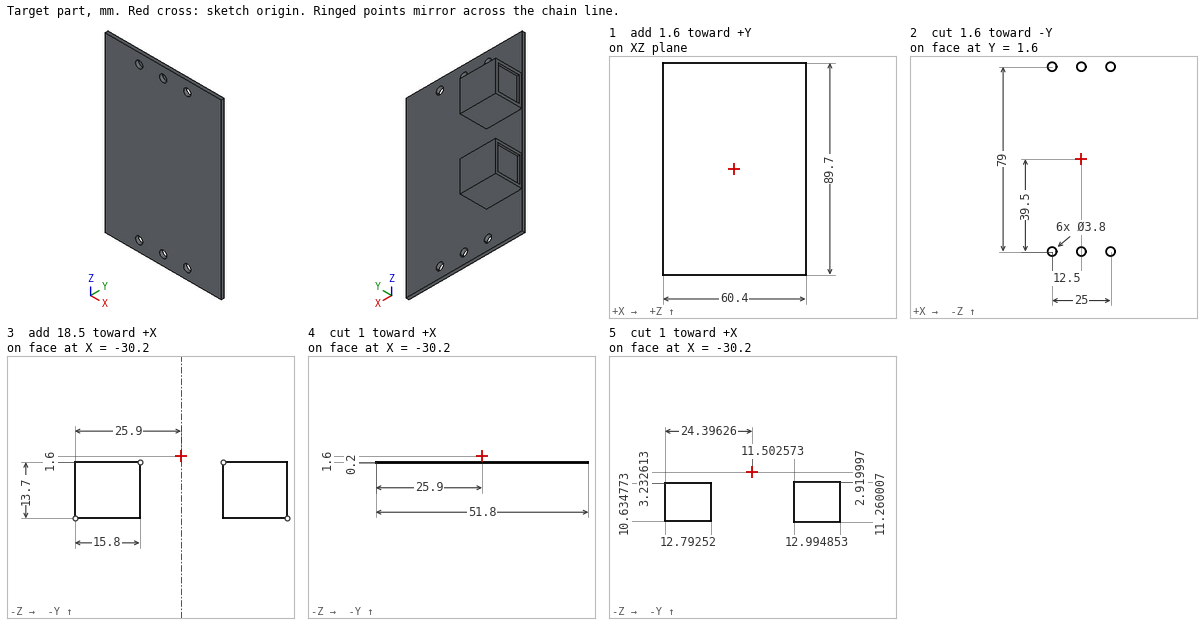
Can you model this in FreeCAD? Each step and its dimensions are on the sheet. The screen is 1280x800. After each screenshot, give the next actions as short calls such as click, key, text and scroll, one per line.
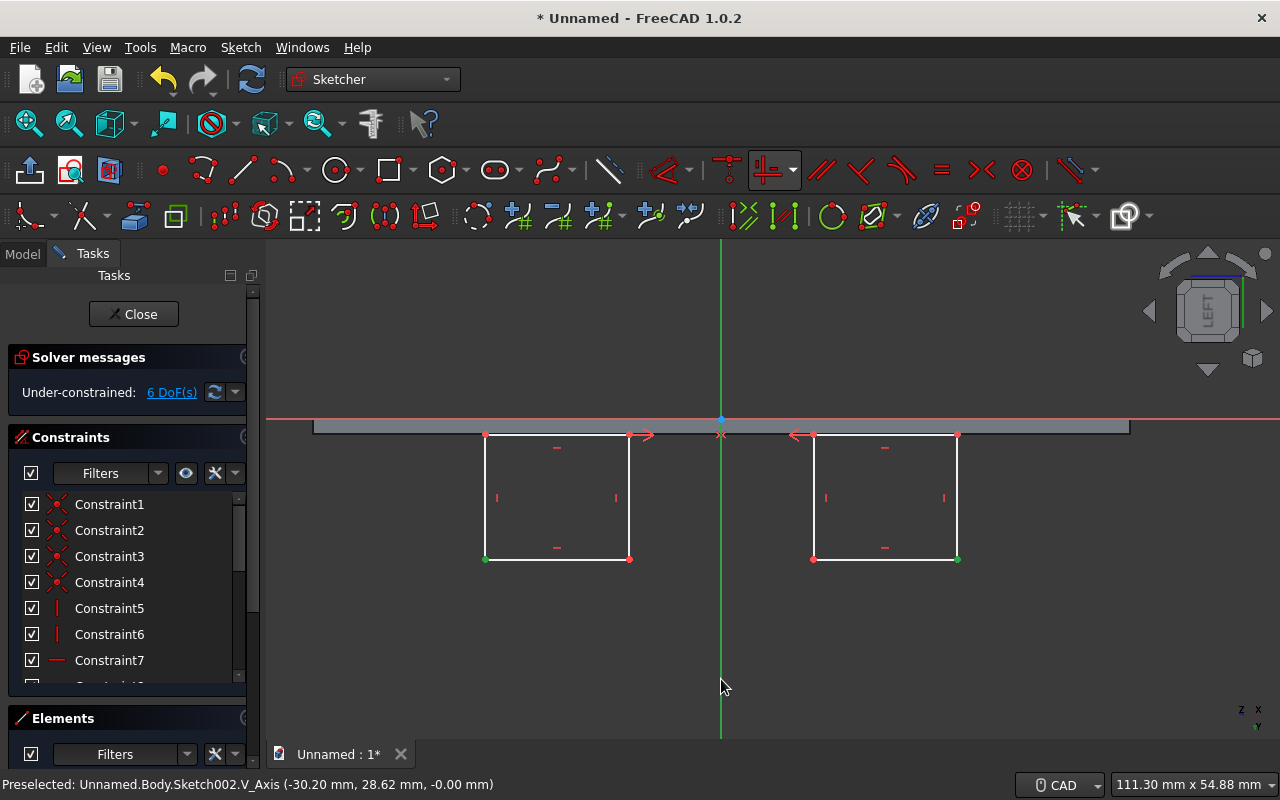
key(s)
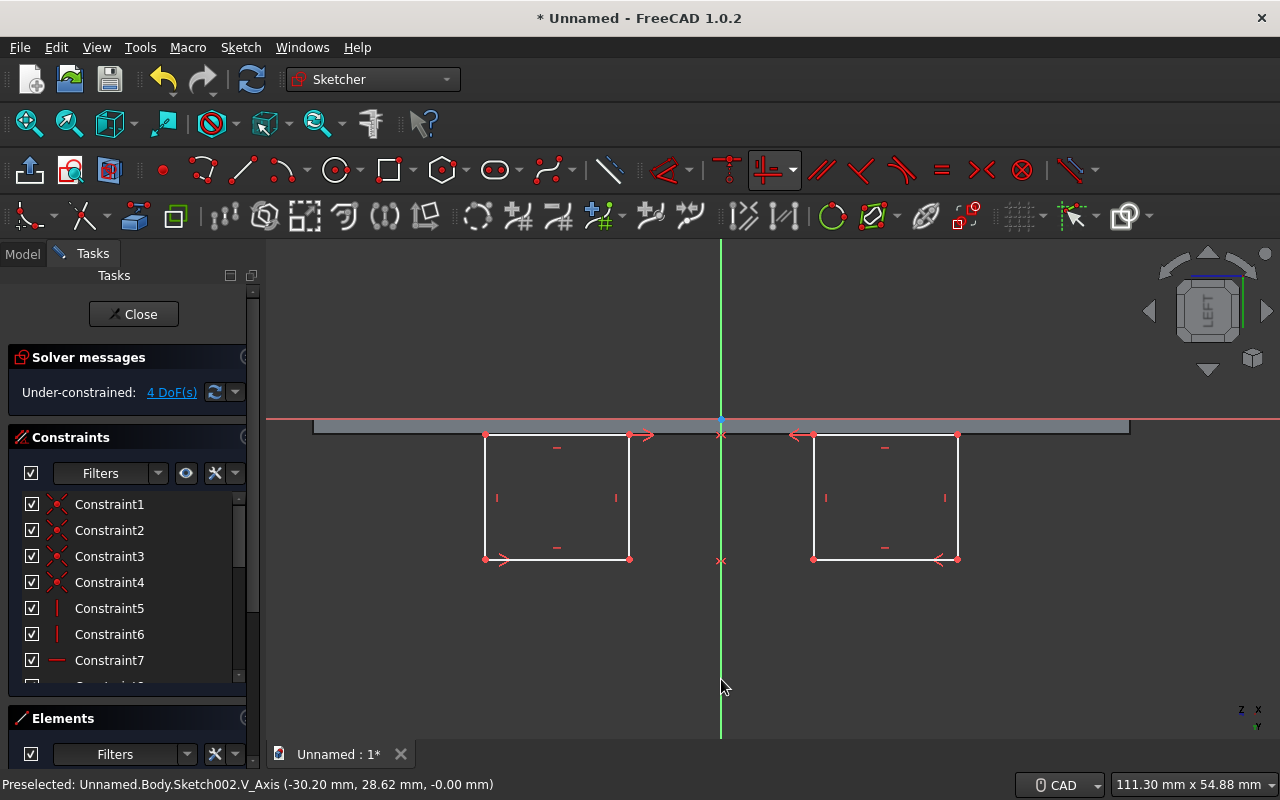
key(d)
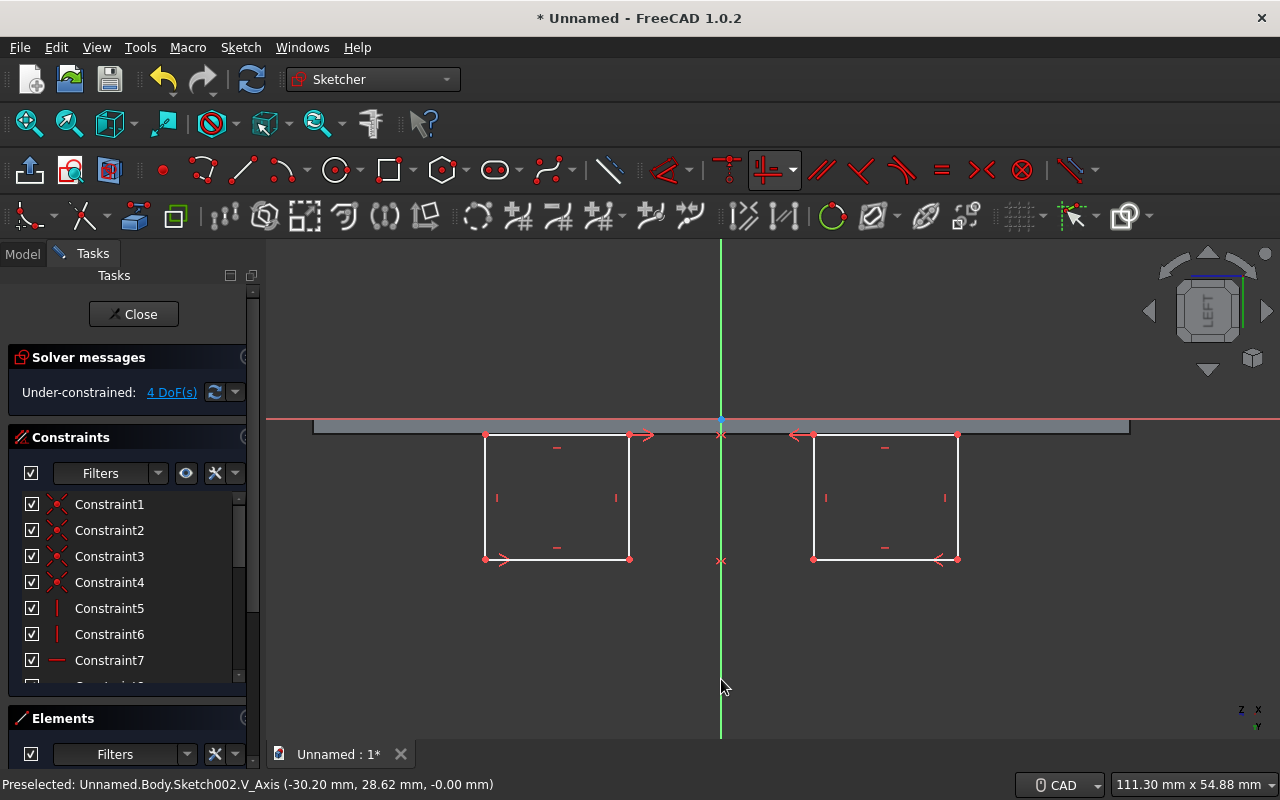
click(485, 473)
click(451, 498)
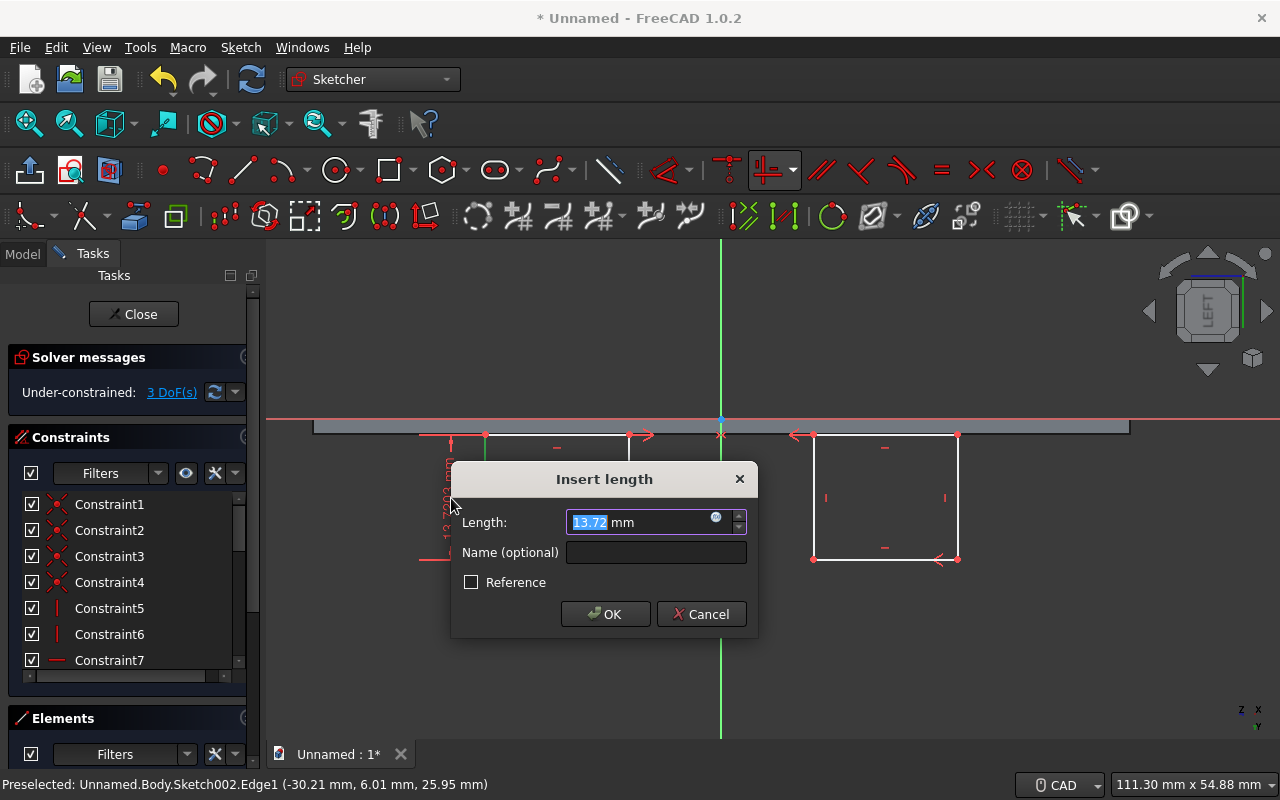
text(13.7)
key(Return)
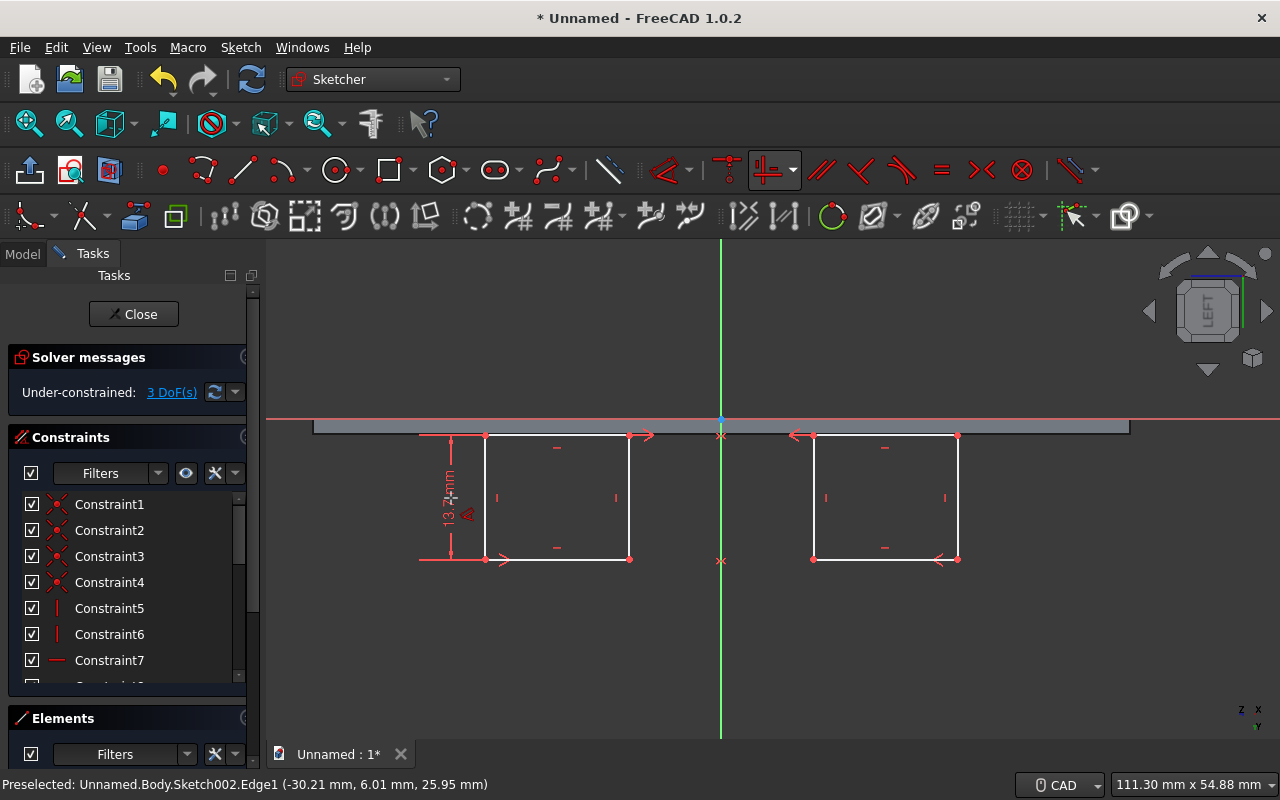
click(528, 560)
click(557, 594)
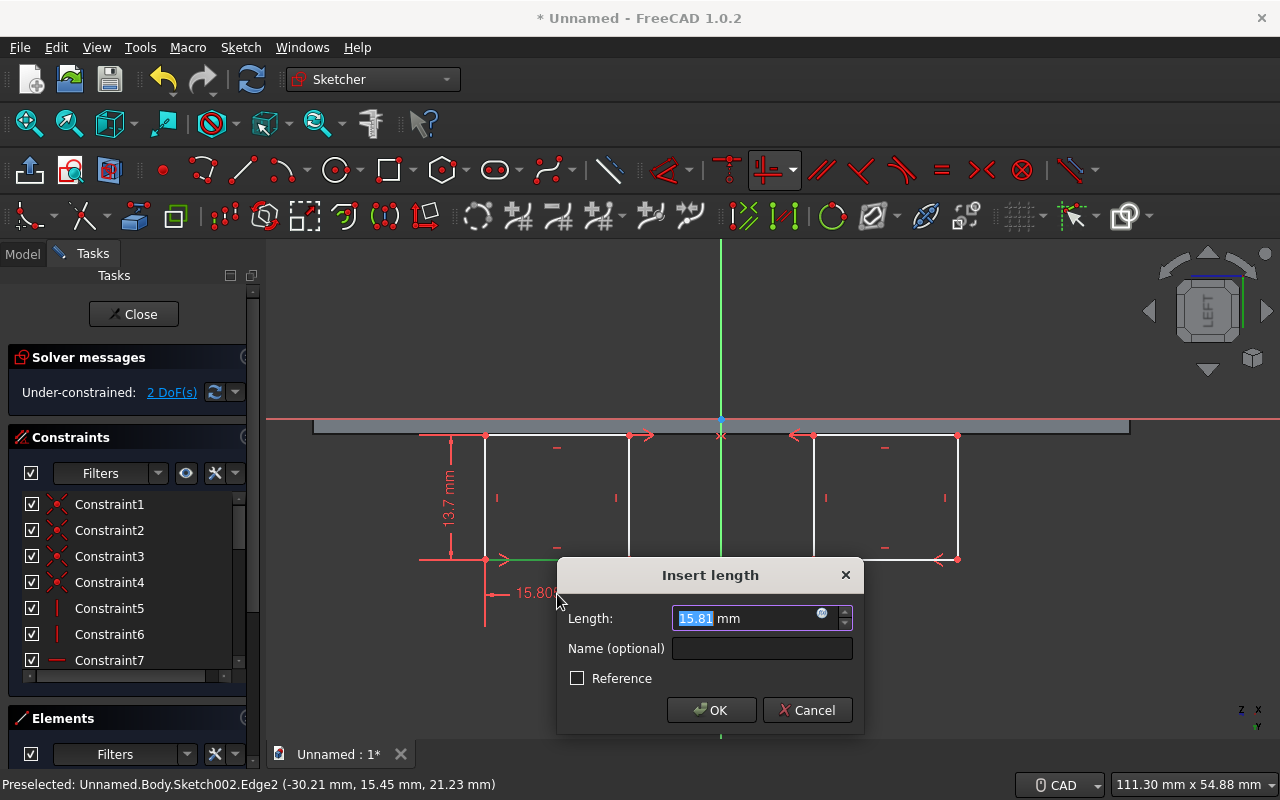
text(15.8)
key(Return)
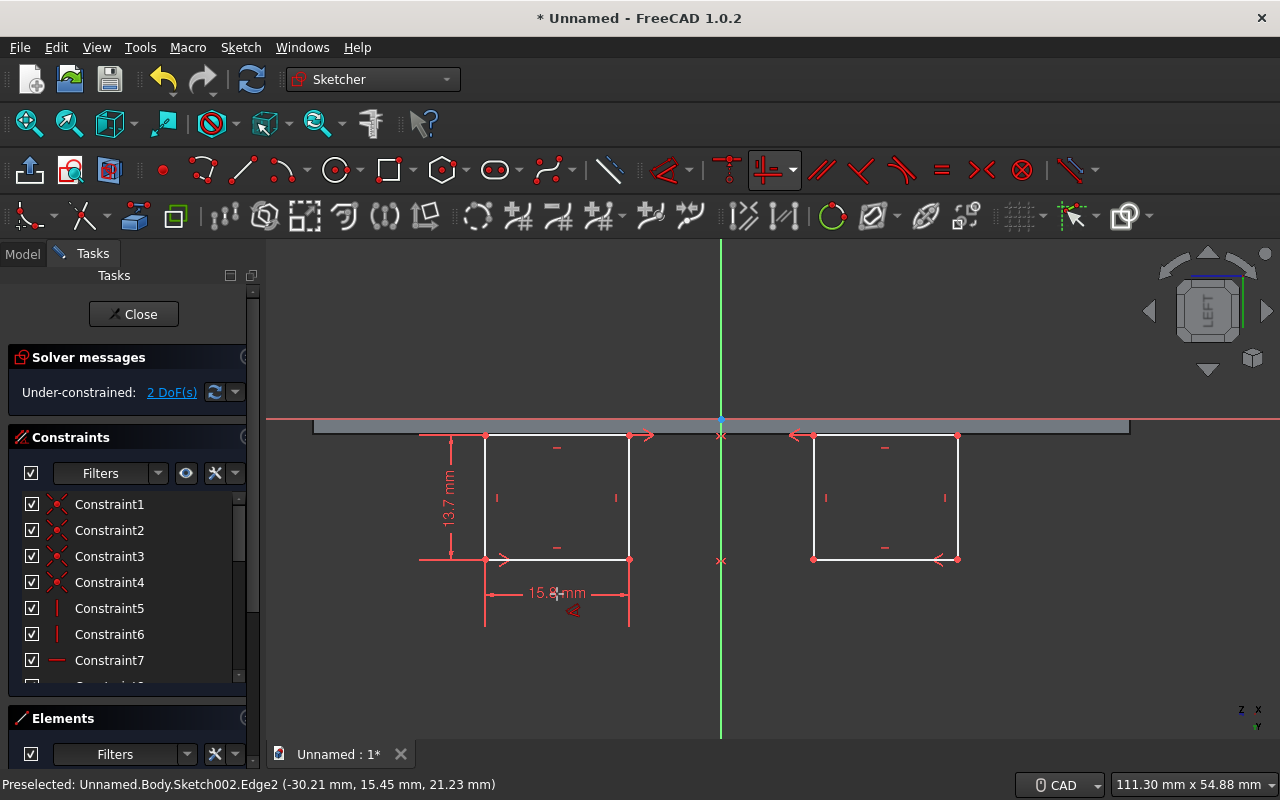
scroll(485, 435, up, 6)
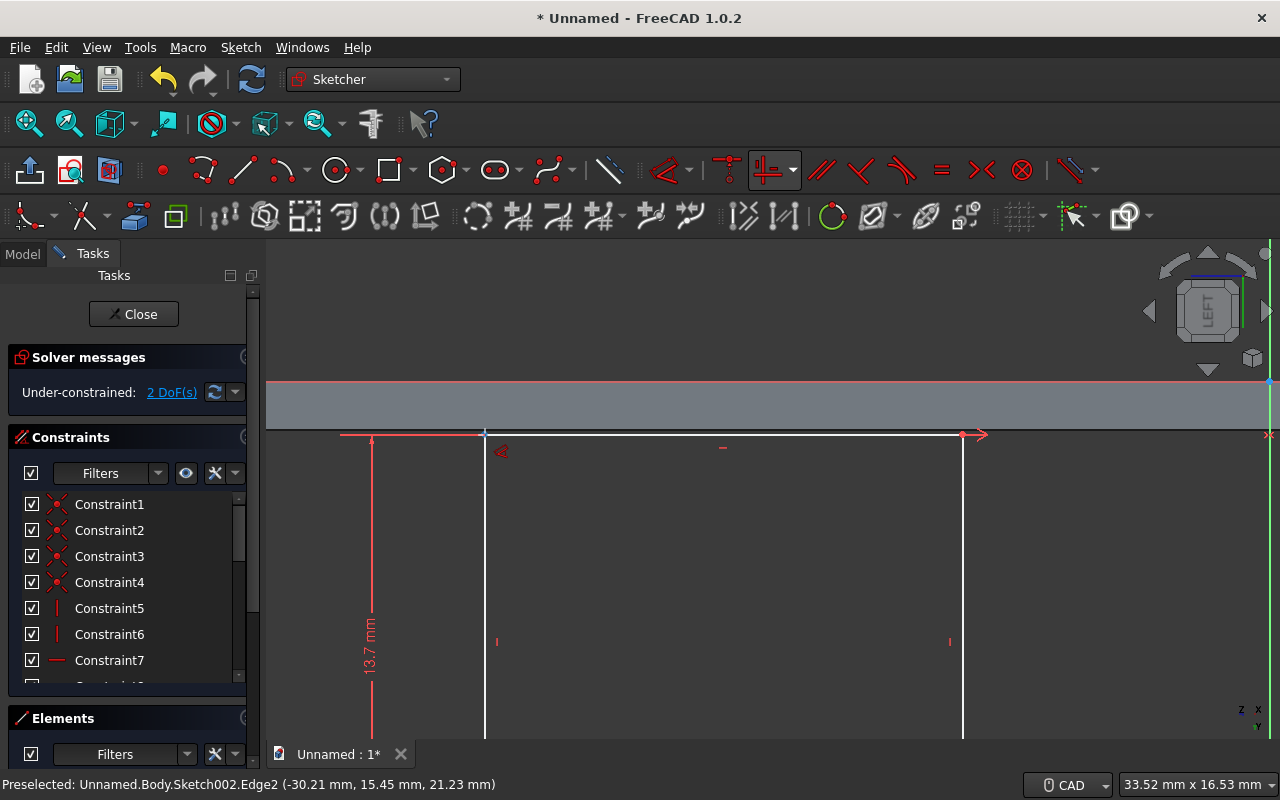
click(485, 435)
click(451, 408)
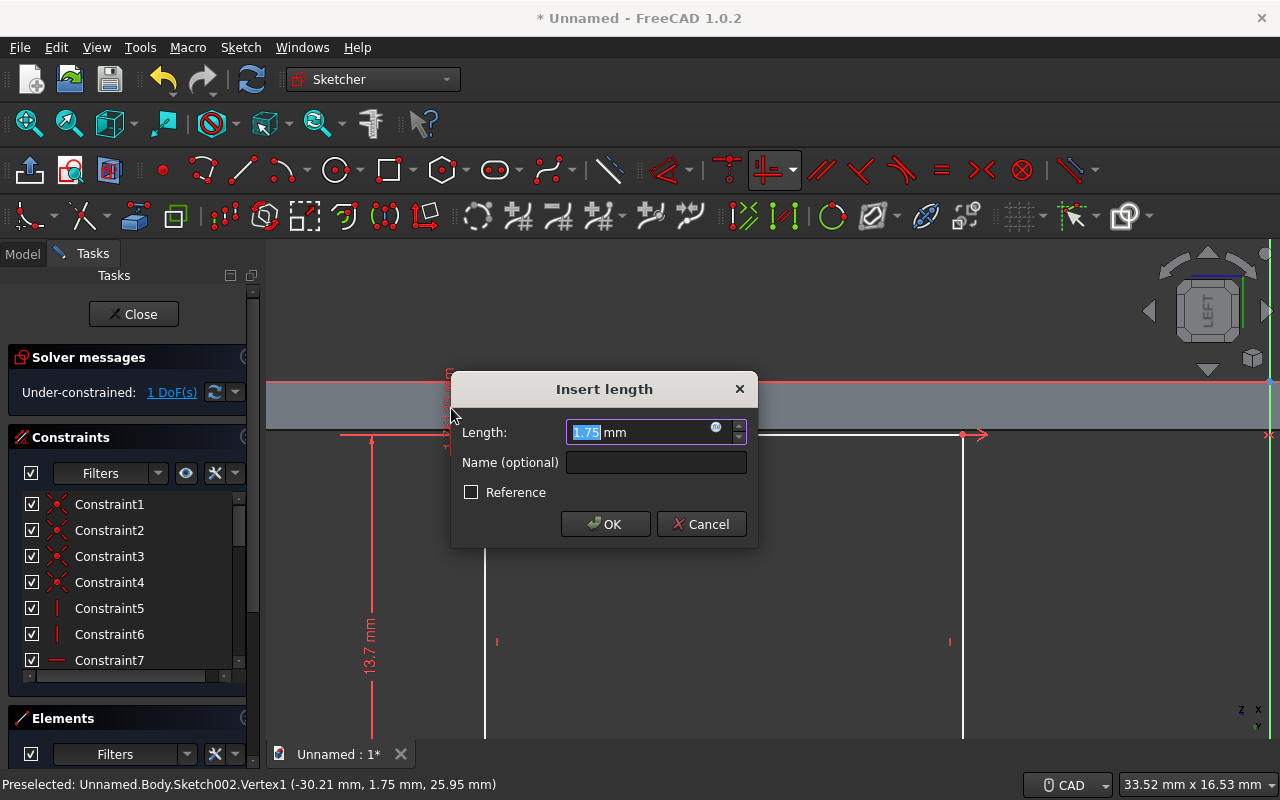
text(1.6)
key(Return)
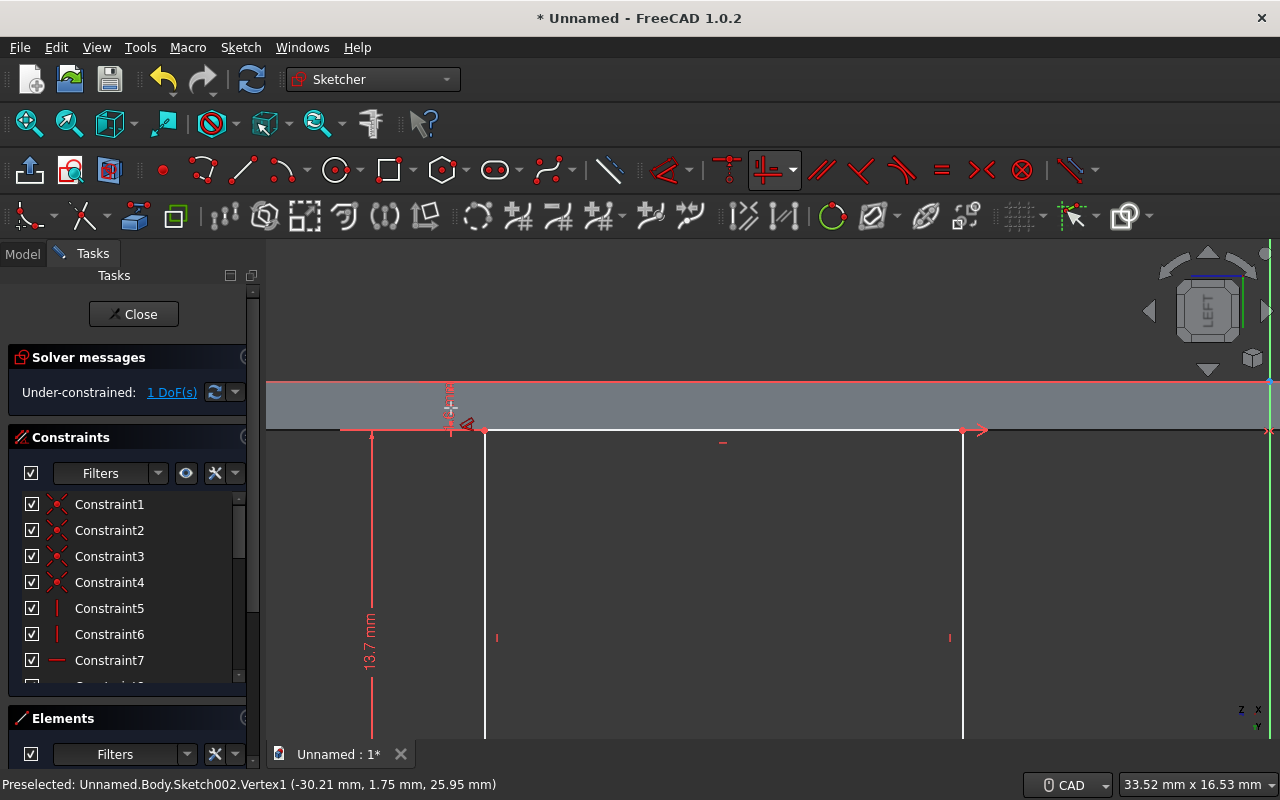
click(485, 430)
click(800, 348)